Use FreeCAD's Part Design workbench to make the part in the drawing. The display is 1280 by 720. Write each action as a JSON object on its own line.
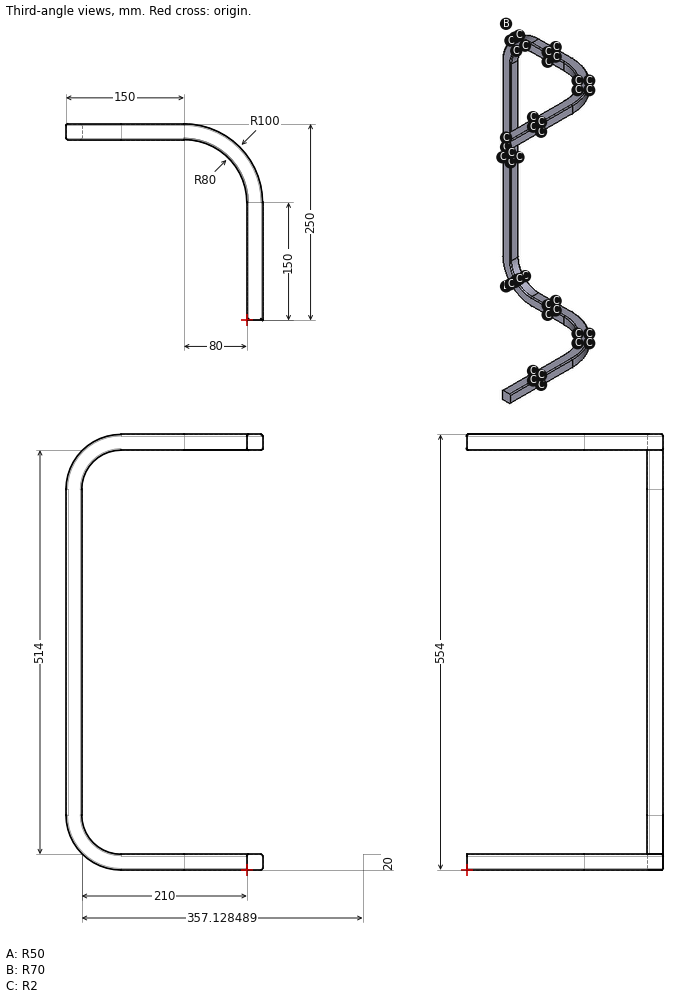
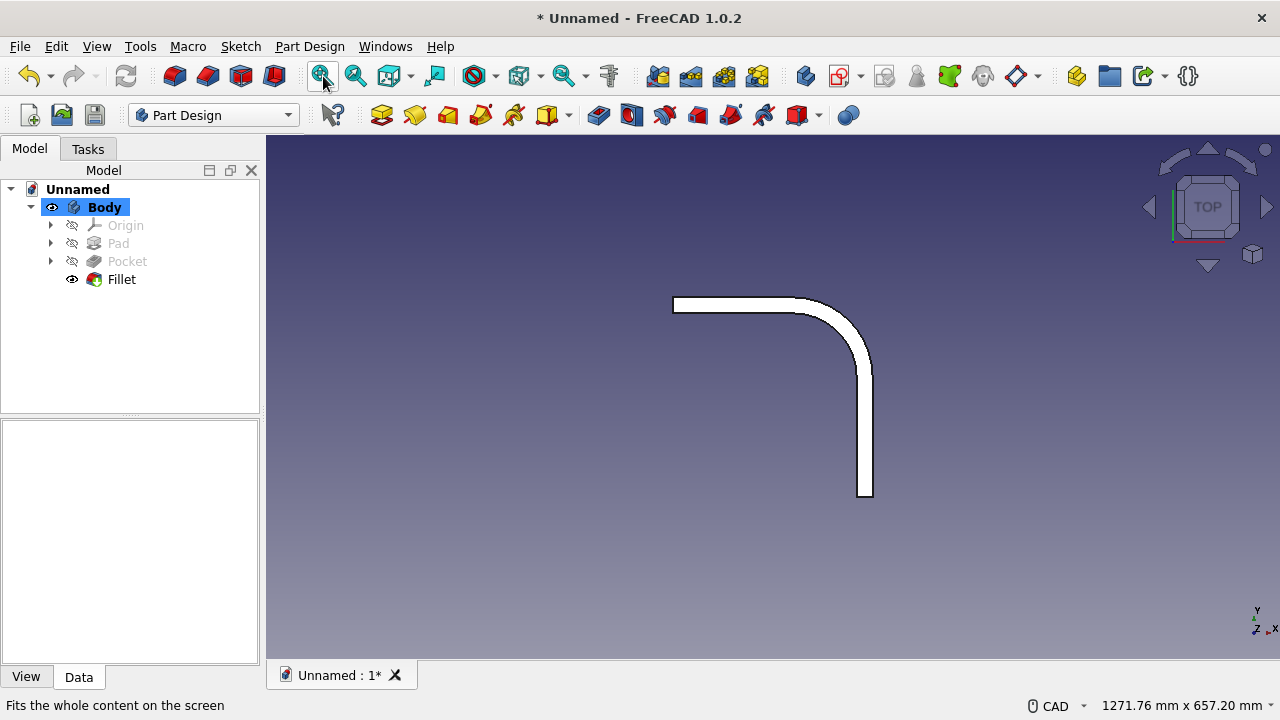
{"action": "left_click", "coordinate": [673, 304]}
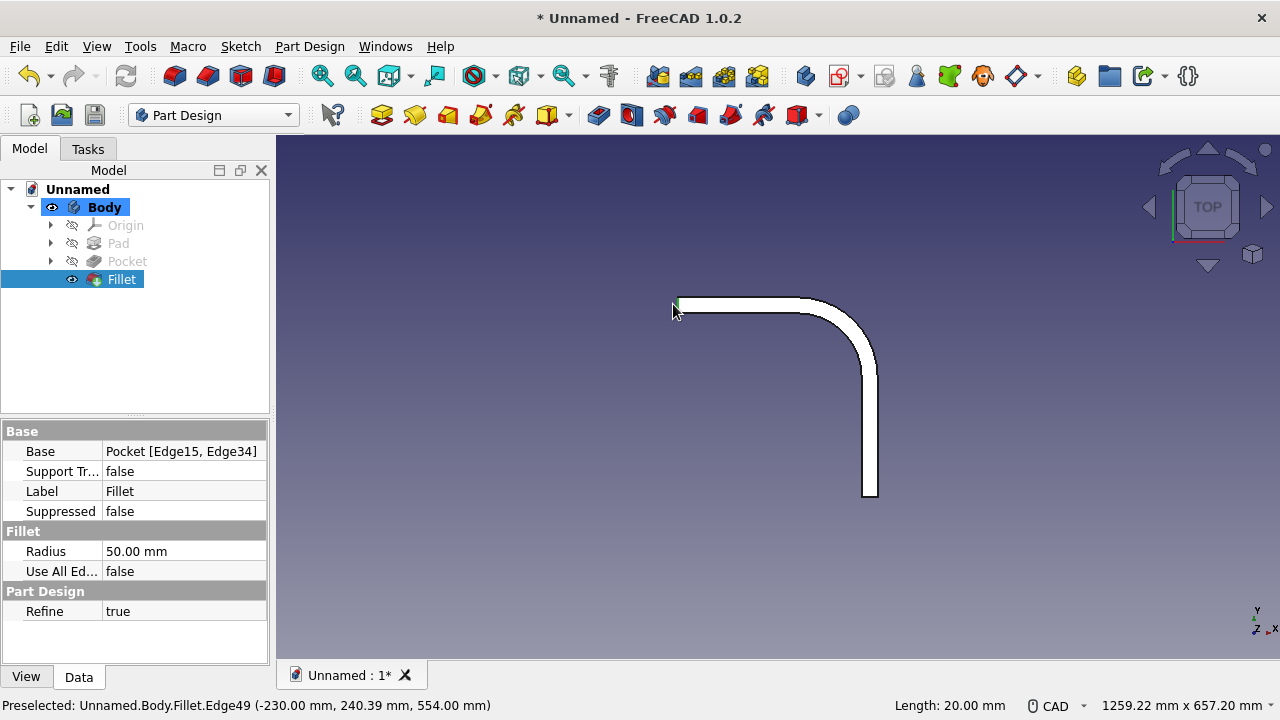
{"action": "scroll", "coordinate": [678, 304], "scroll_direction": "up", "scroll_amount": 5}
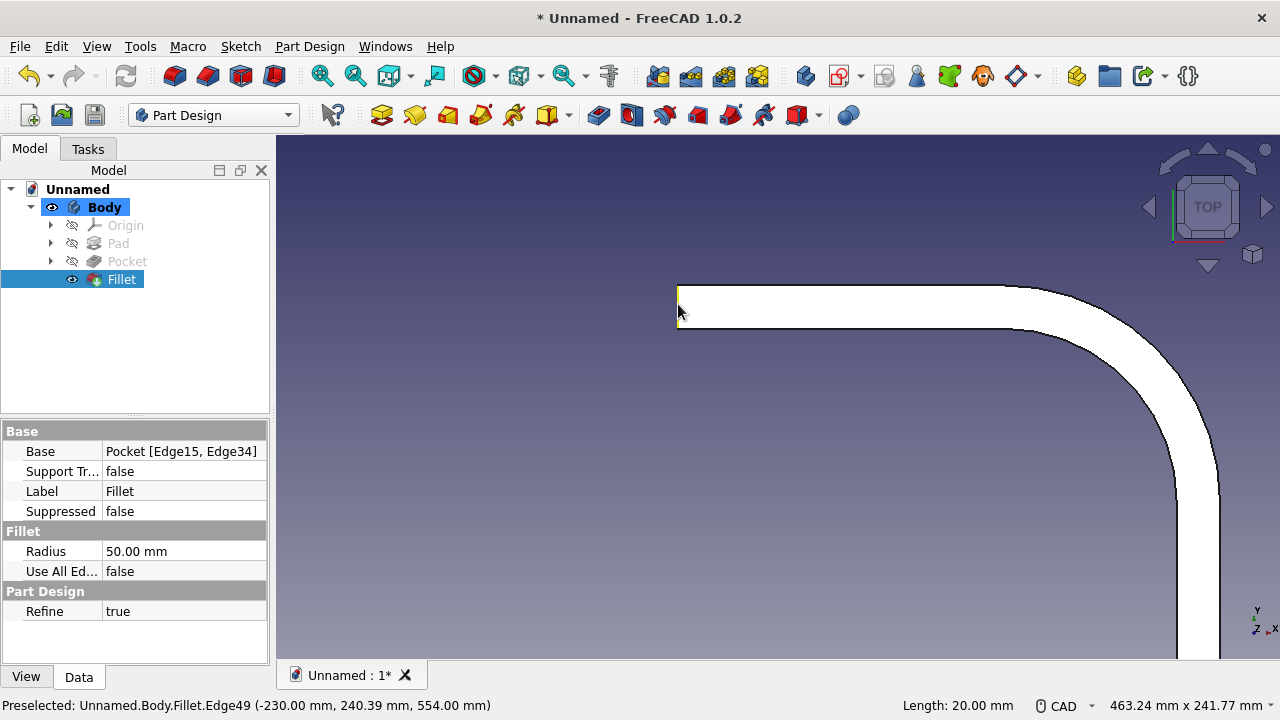
{"action": "left_click", "coordinate": [323, 76]}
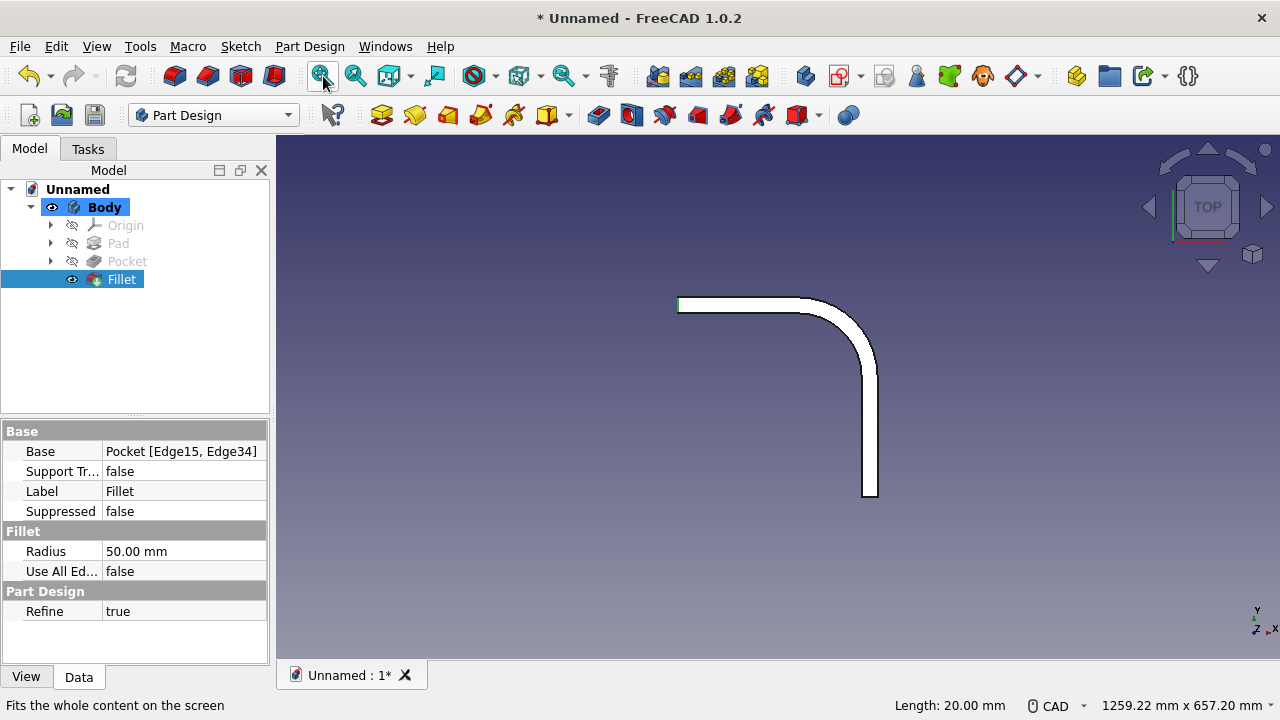
{"action": "key", "text": "0"}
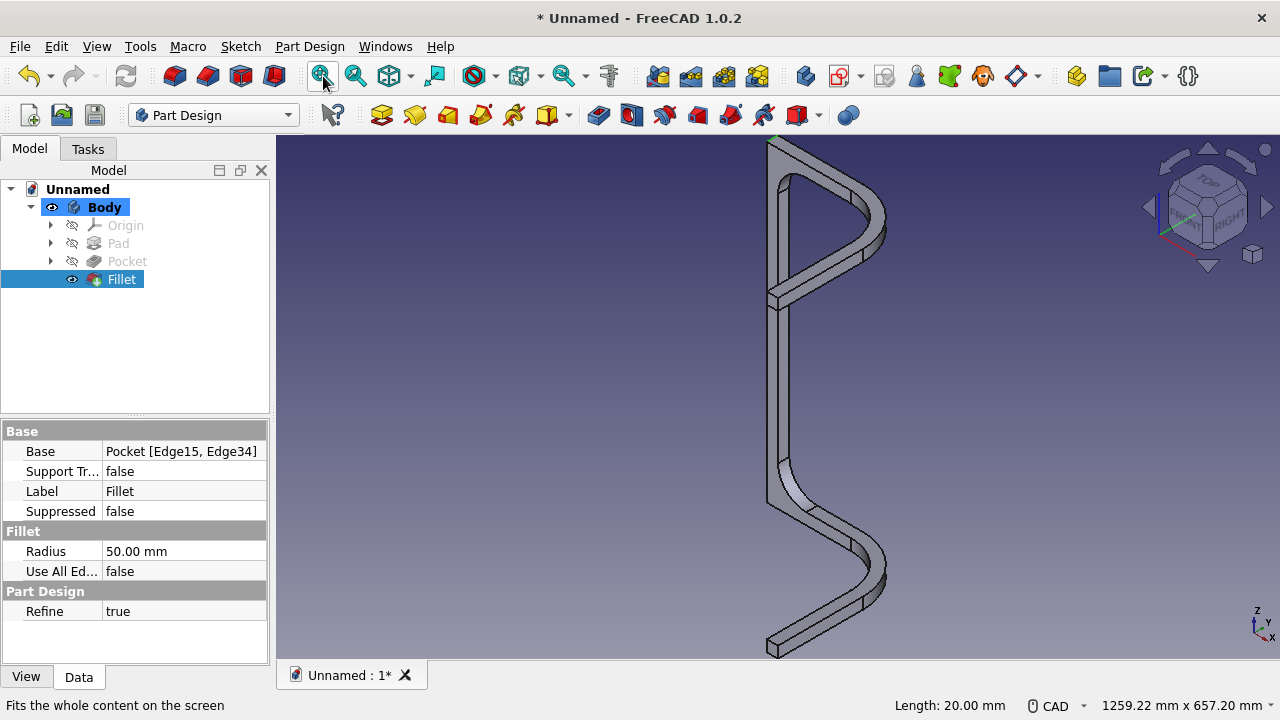
{"action": "left_click", "coordinate": [323, 76]}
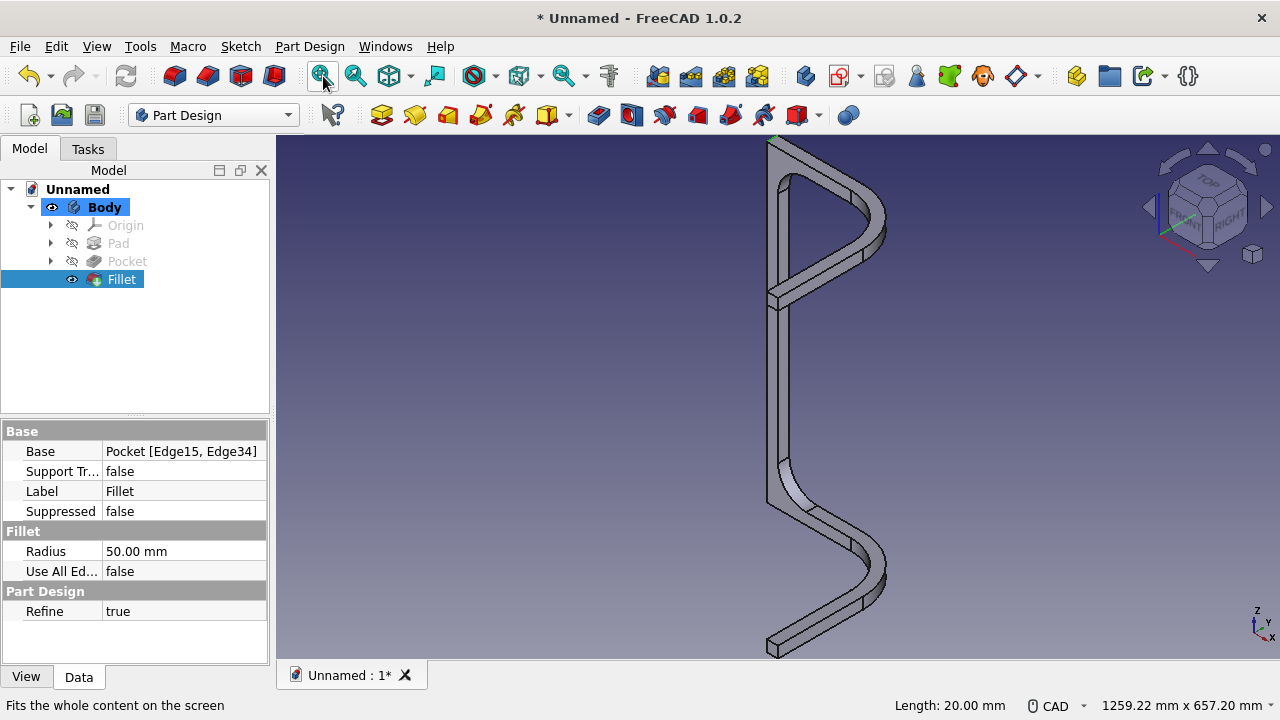
{"action": "scroll", "coordinate": [772, 498], "scroll_direction": "up", "scroll_amount": 5}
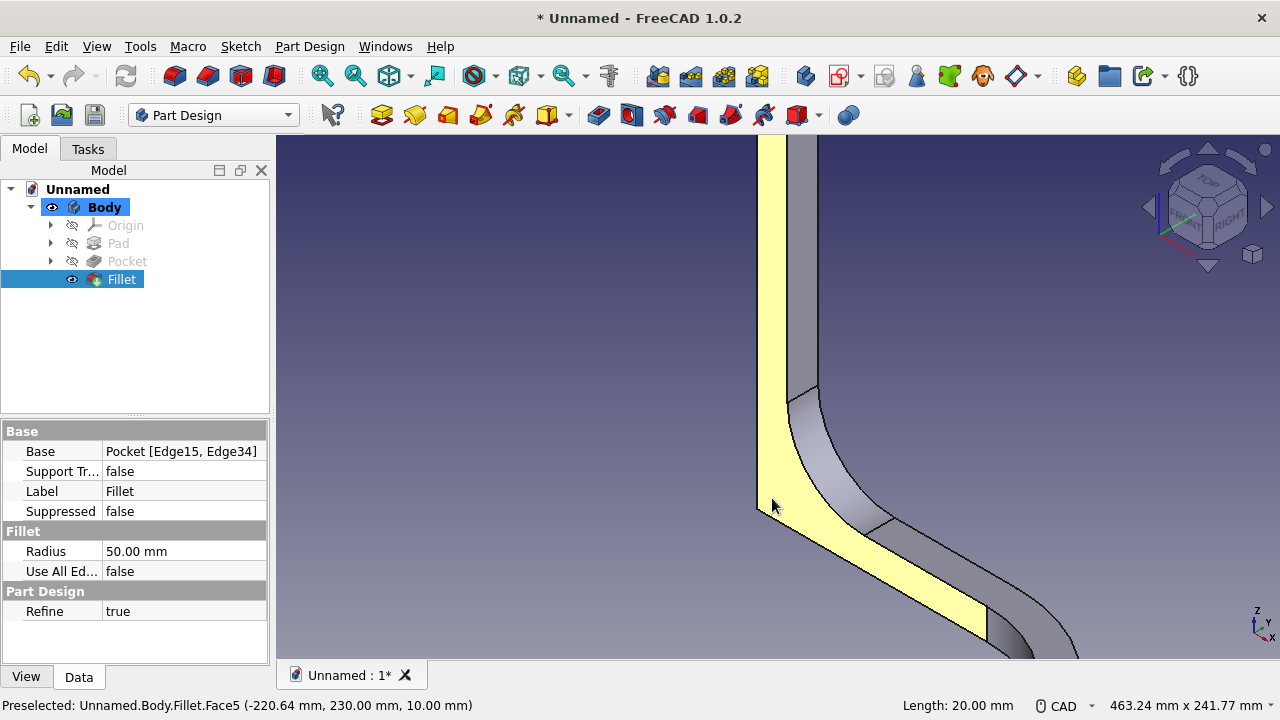
{"action": "left_click", "coordinate": [323, 76]}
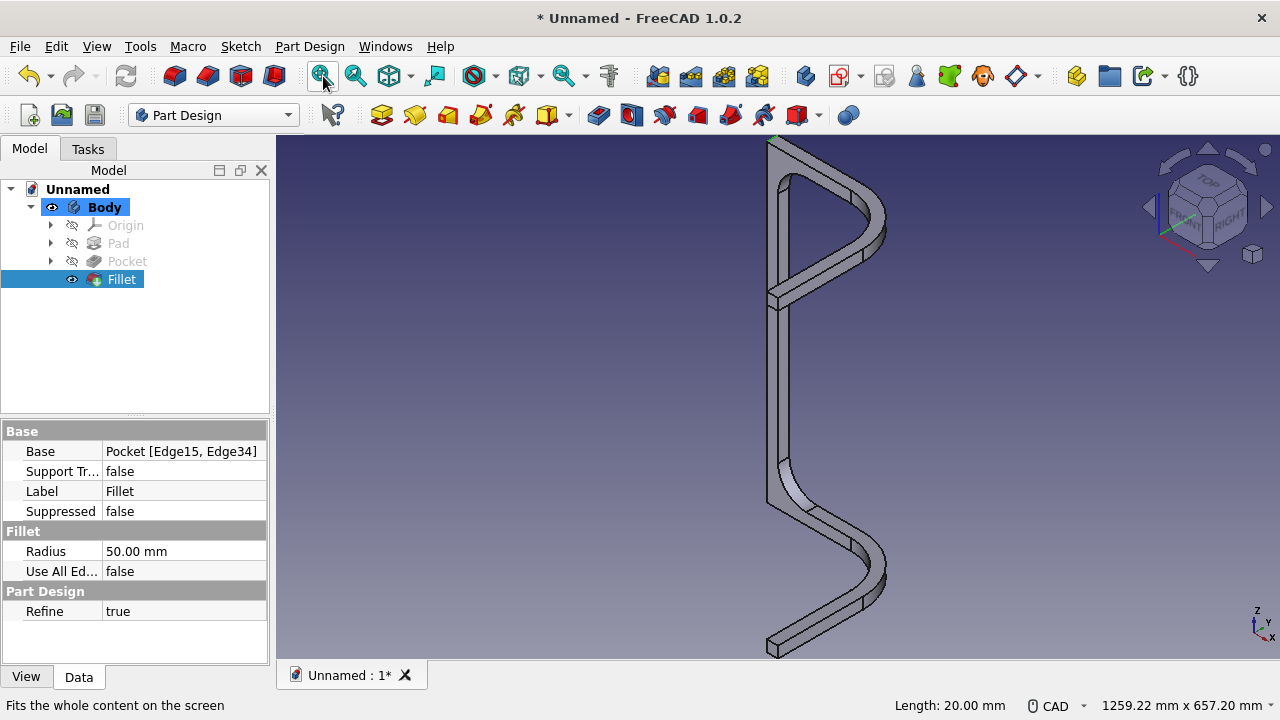
{"action": "key", "text": "2"}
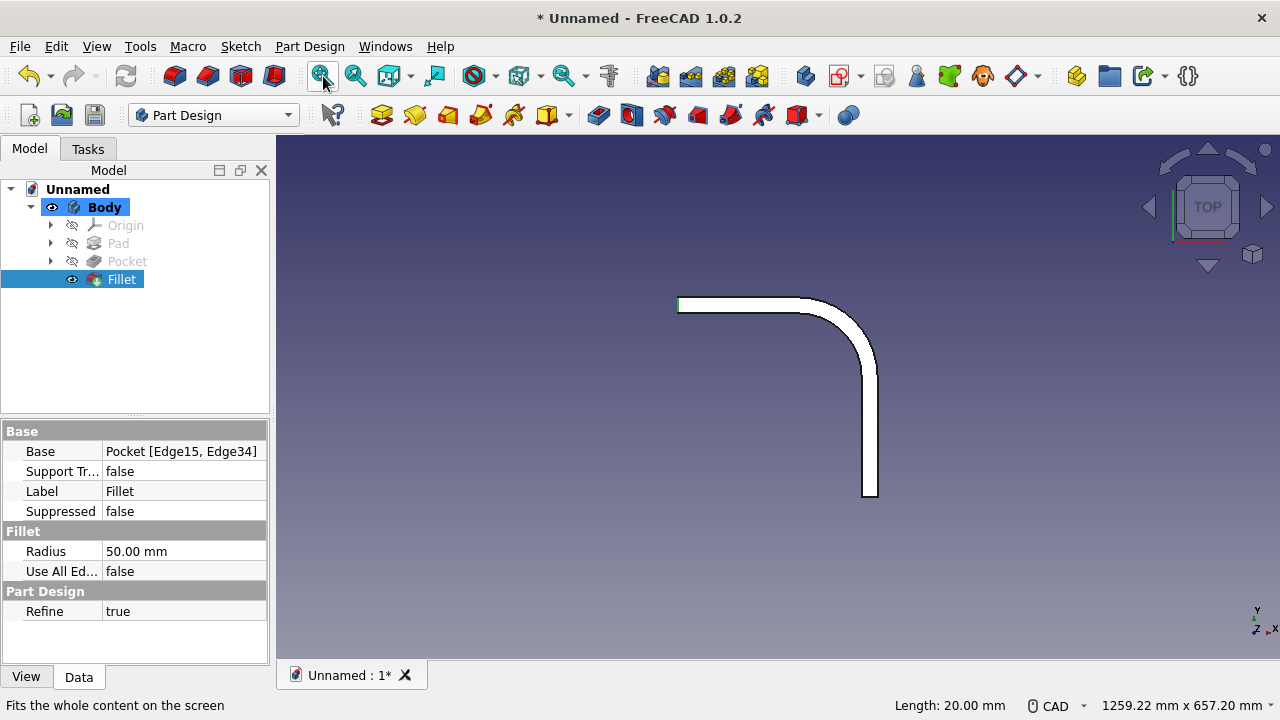
{"action": "left_click", "coordinate": [323, 76]}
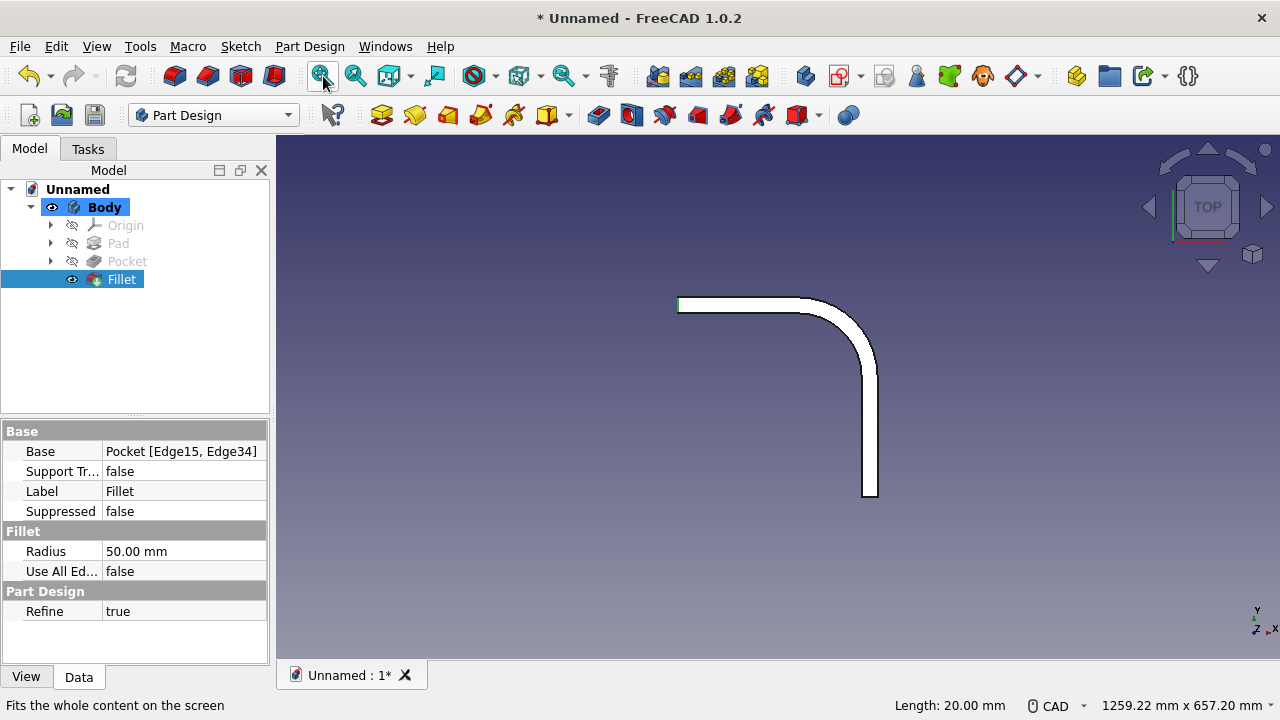
{"action": "scroll", "coordinate": [678, 304], "scroll_direction": "up", "scroll_amount": 5}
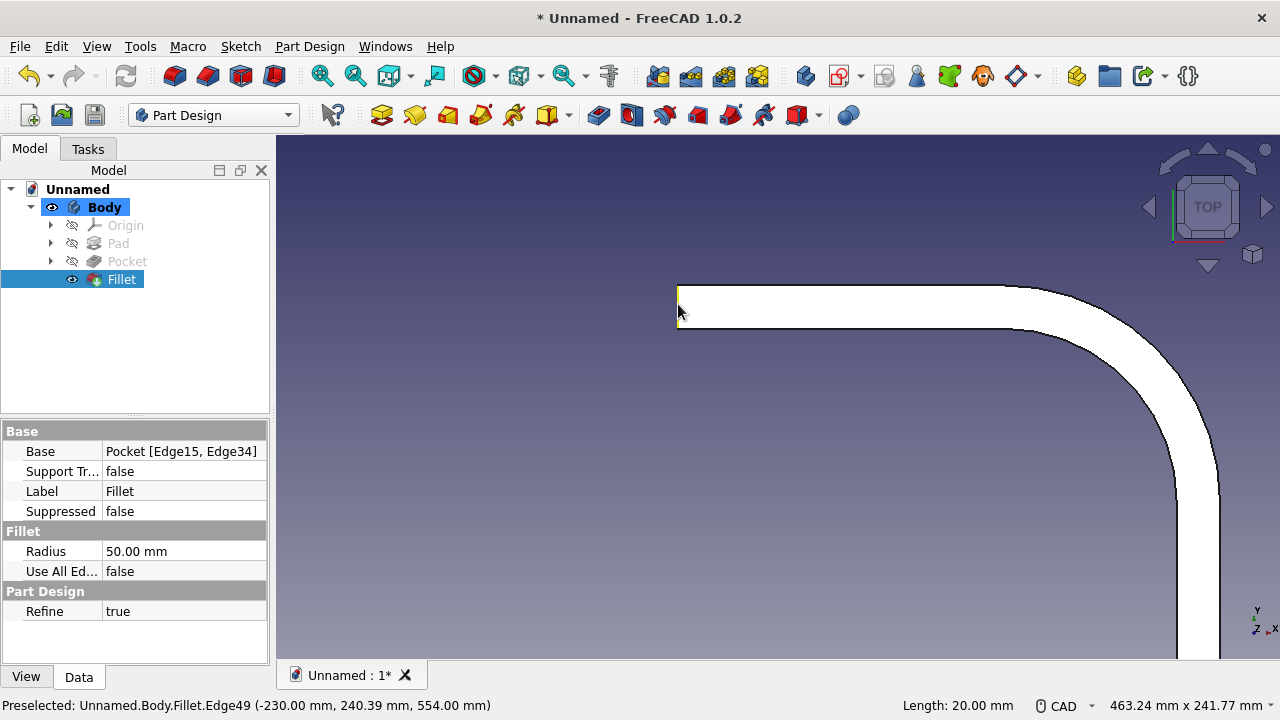
{"action": "left_click", "coordinate": [323, 76]}